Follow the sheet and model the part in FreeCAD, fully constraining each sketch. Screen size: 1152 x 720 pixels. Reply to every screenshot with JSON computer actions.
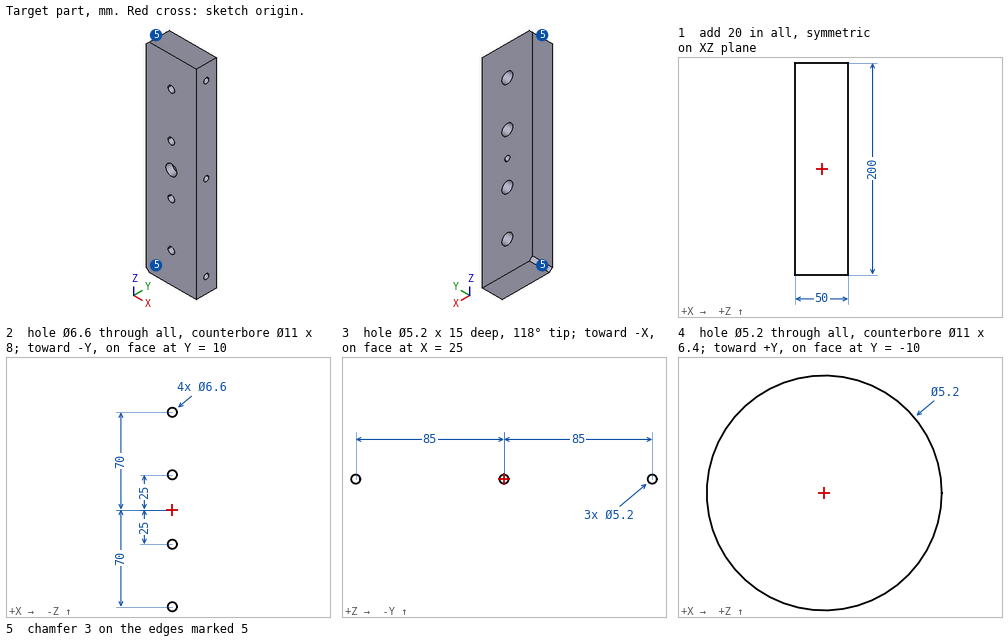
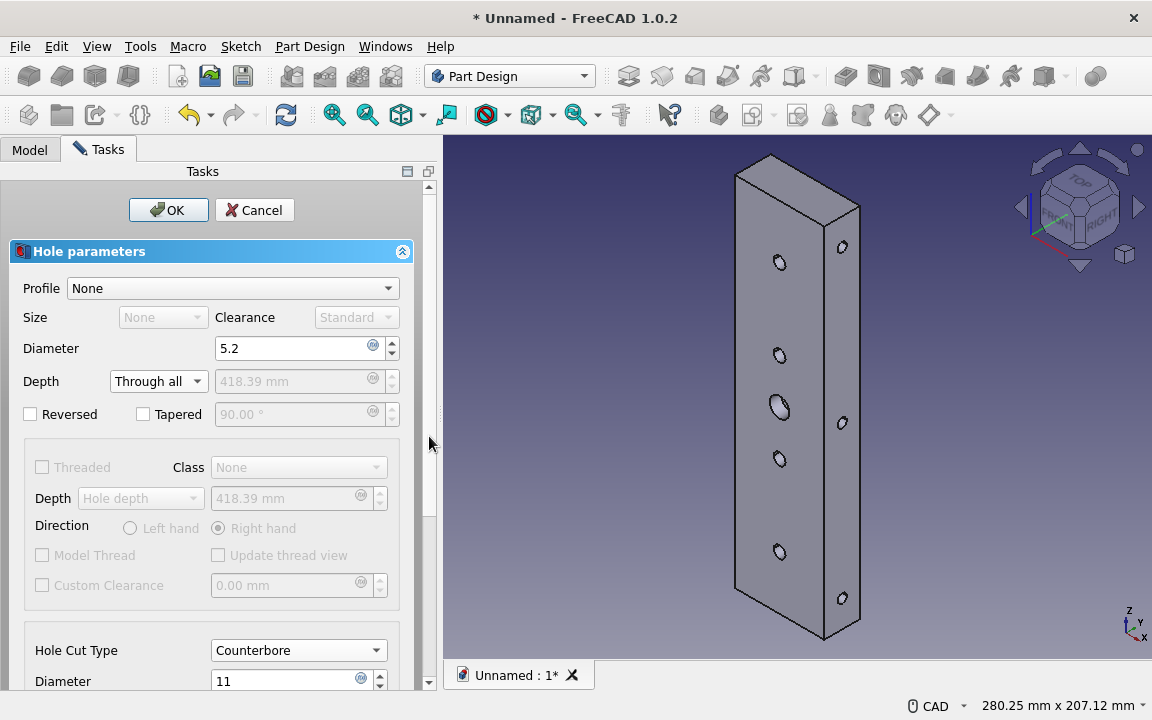
{"action": "left_click", "coordinate": [169, 210]}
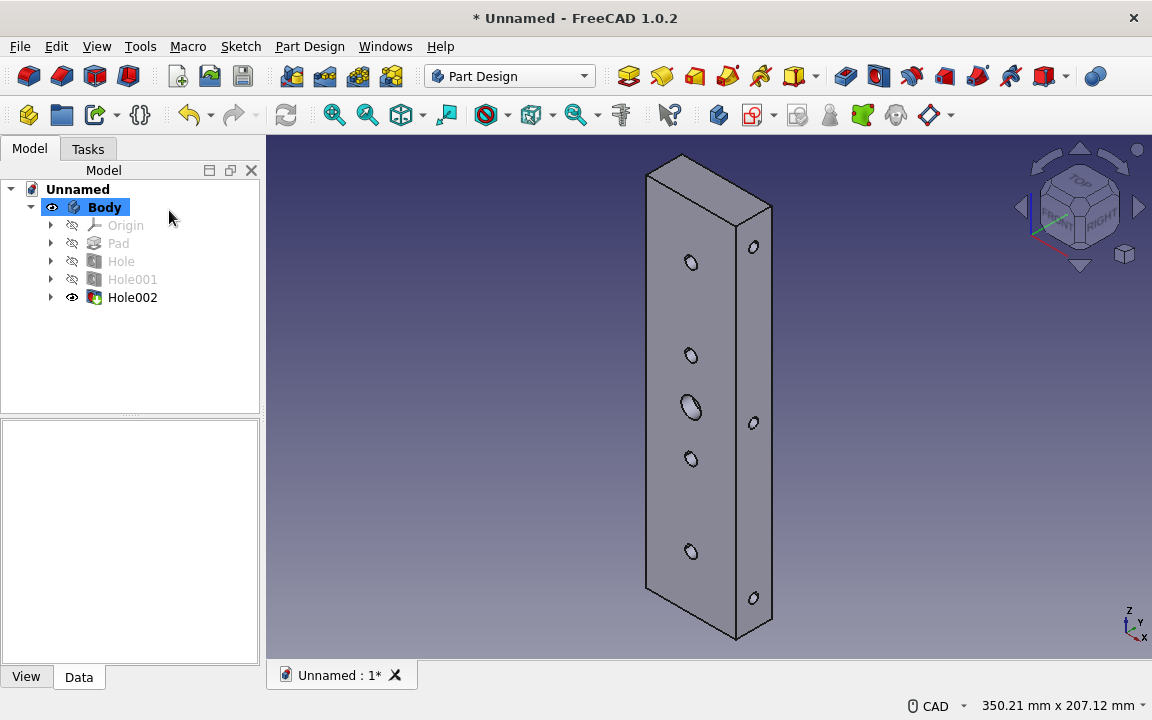
{"action": "key", "text": "2"}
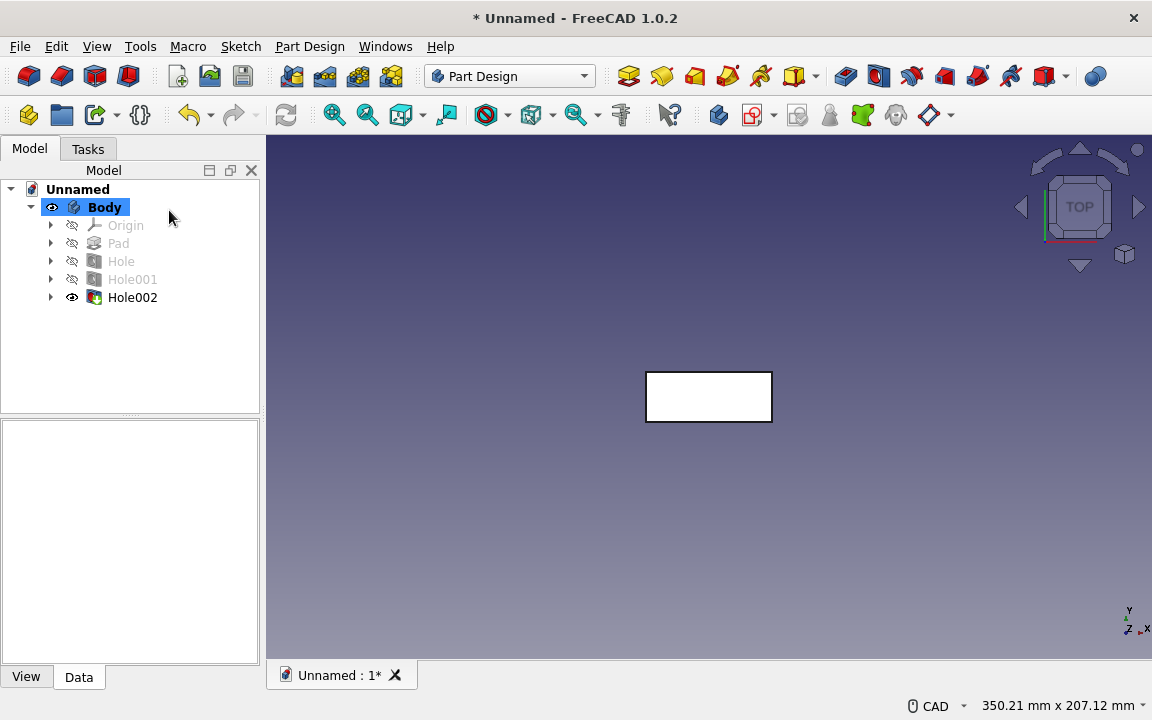
{"action": "left_click", "coordinate": [335, 116]}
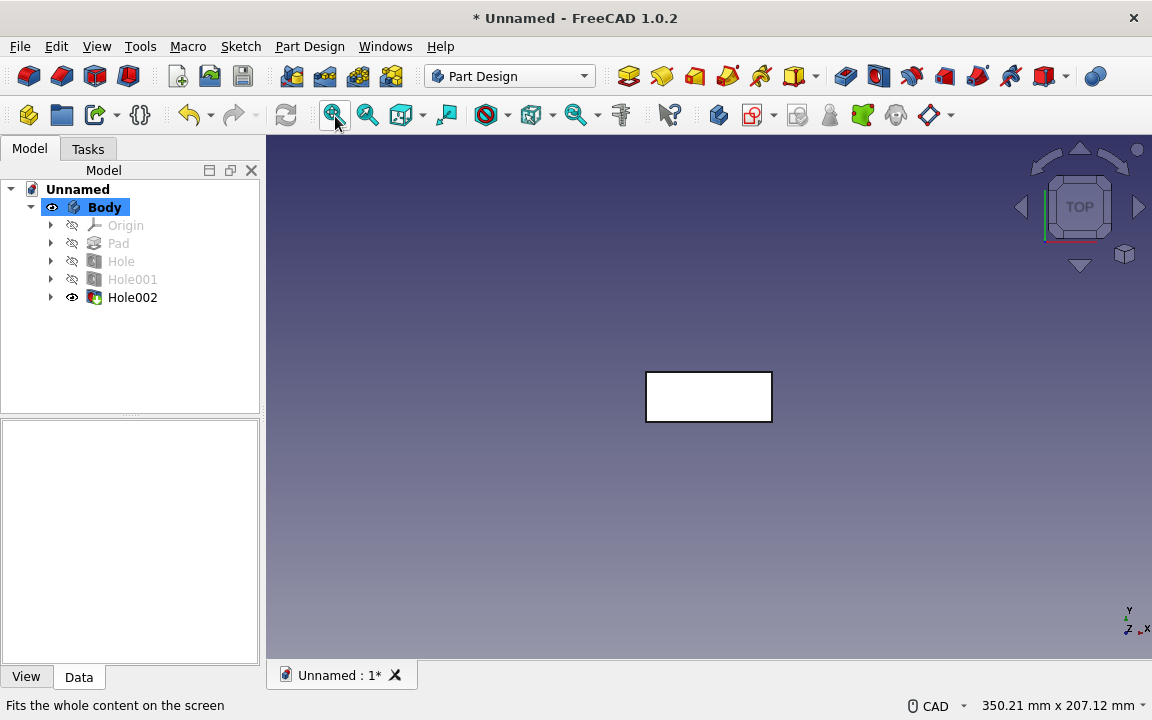
{"action": "left_click", "coordinate": [646, 396]}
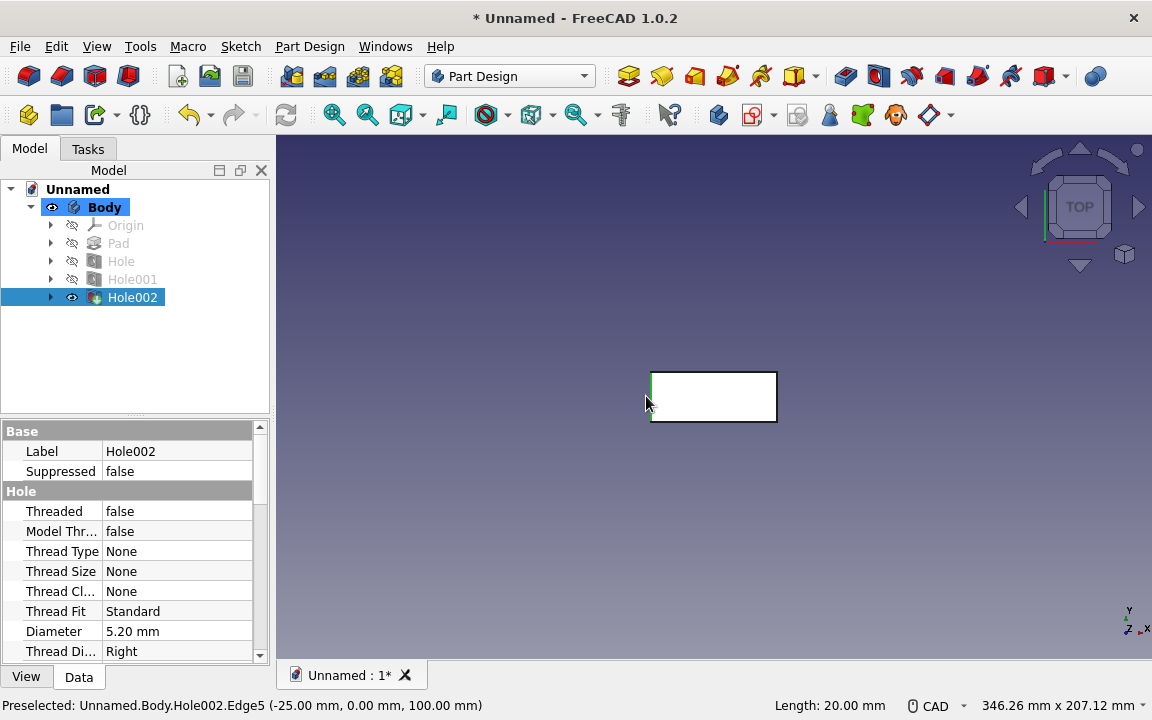
{"action": "key", "text": "0"}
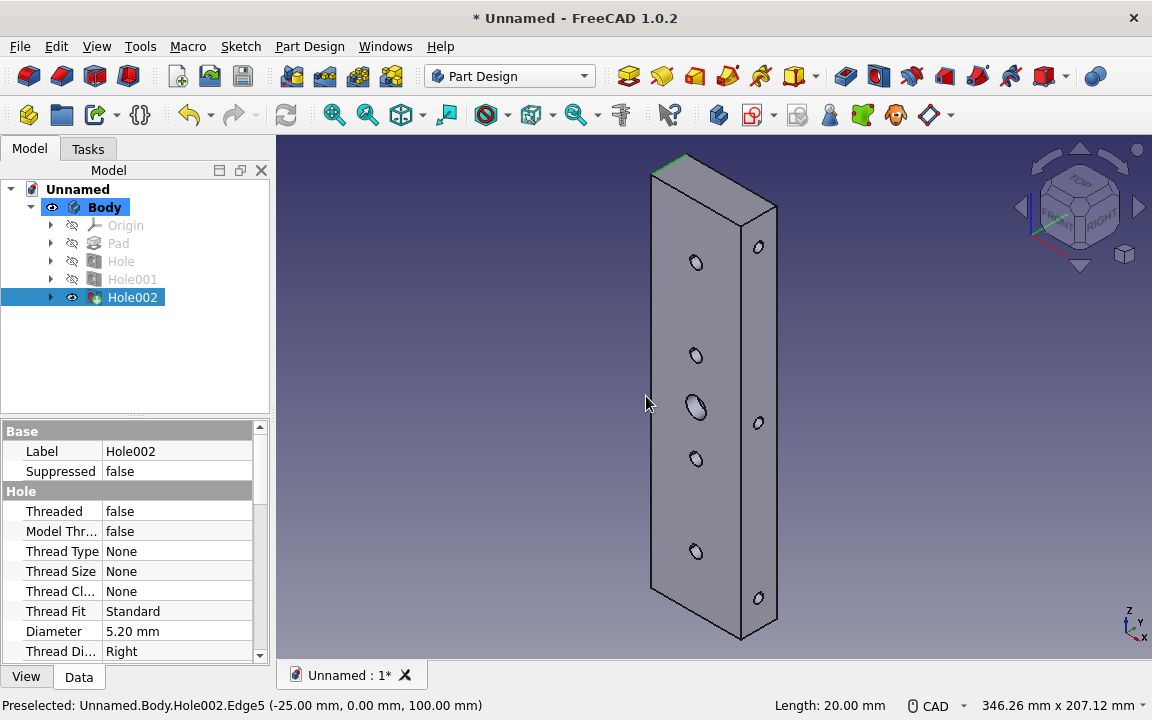
{"action": "key", "text": "1"}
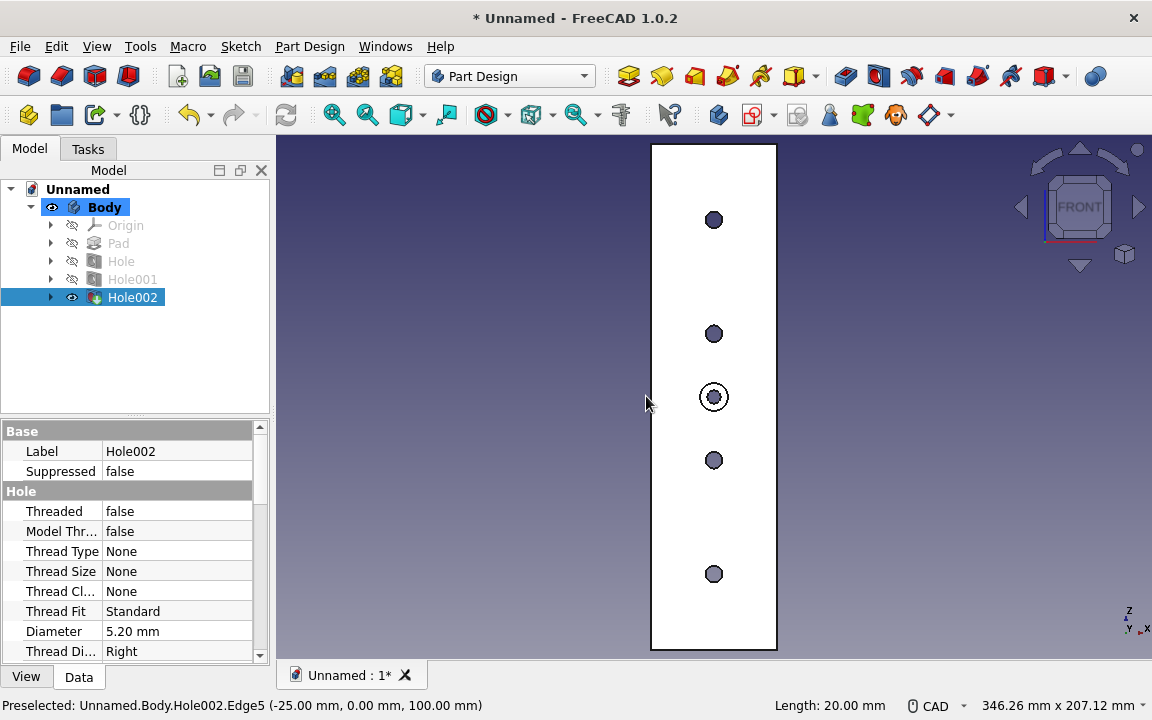
{"action": "key", "text": "3"}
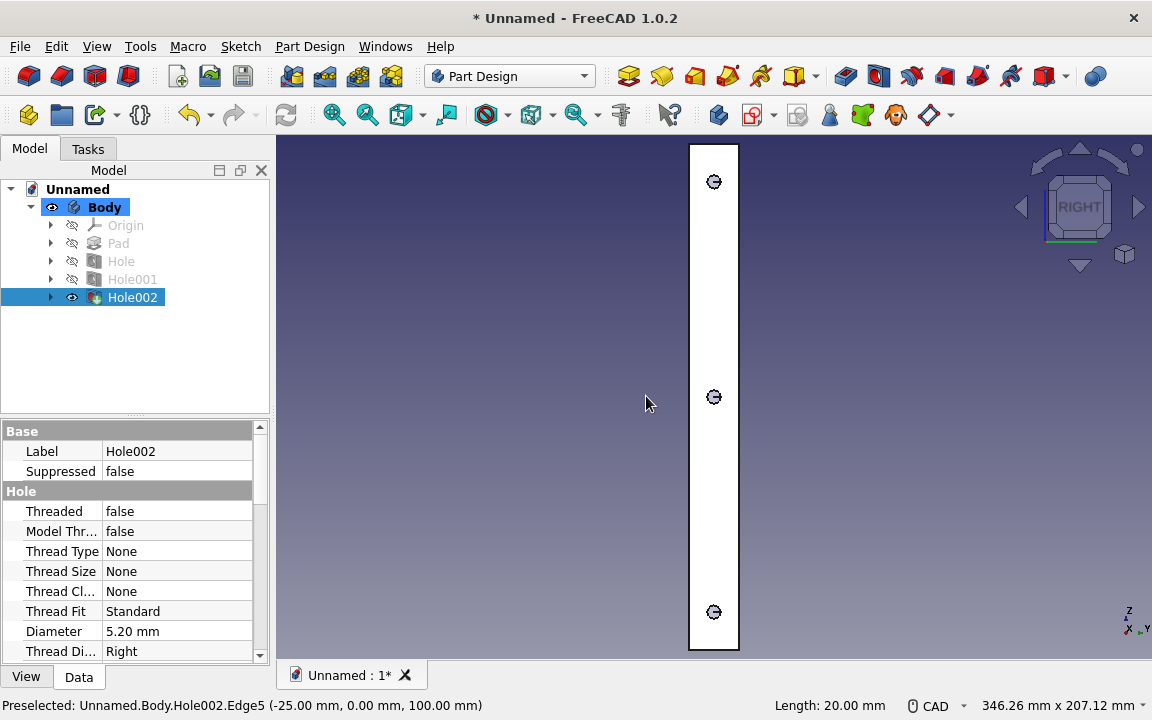
{"action": "key", "text": "5"}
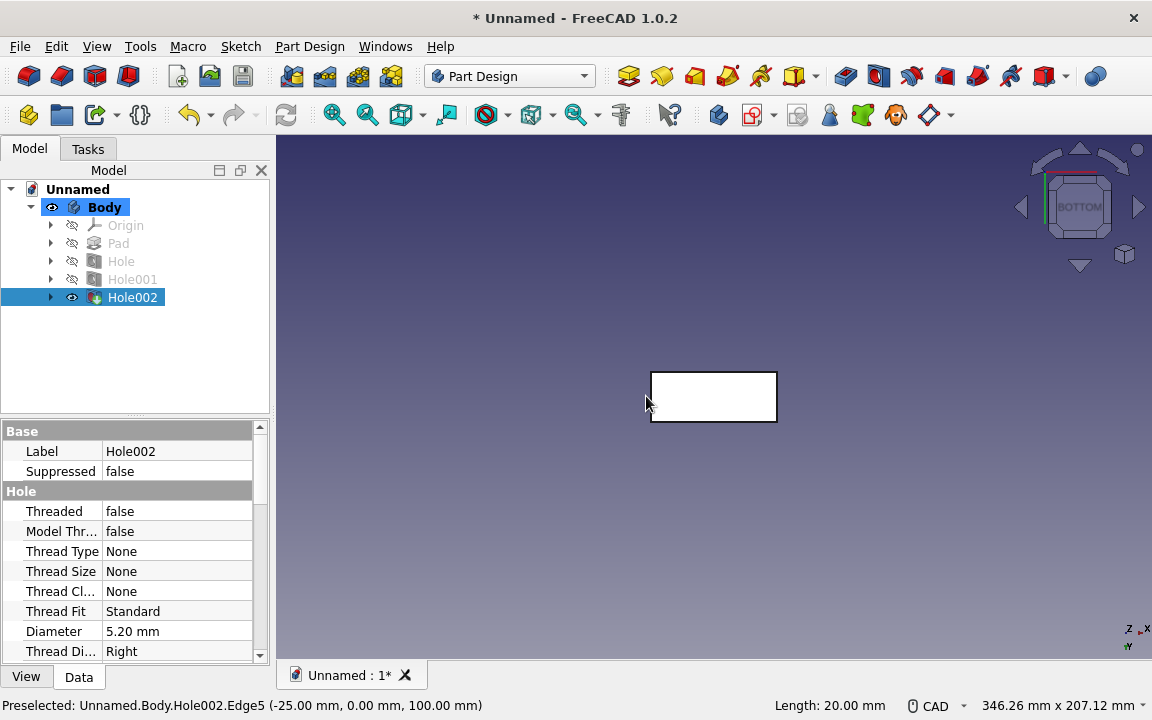
{"action": "left_click", "coordinate": [335, 116]}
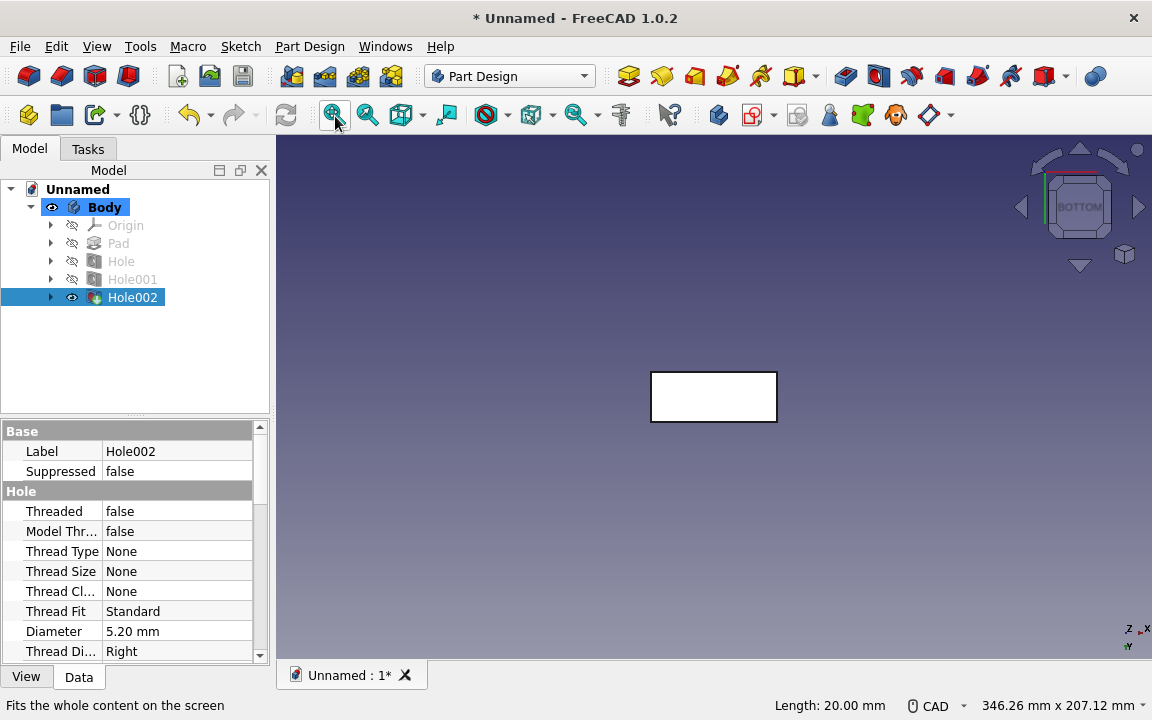
{"action": "left_click", "coordinate": [651, 396], "text": "ctrl"}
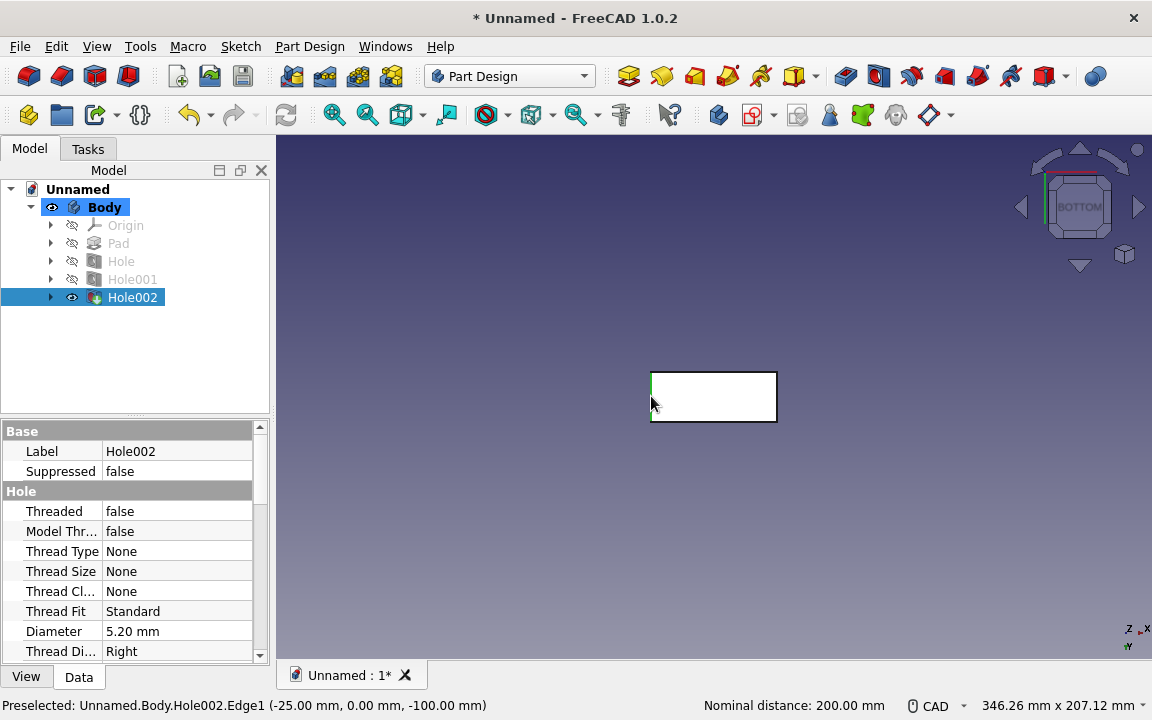
{"action": "left_click", "coordinate": [62, 76]}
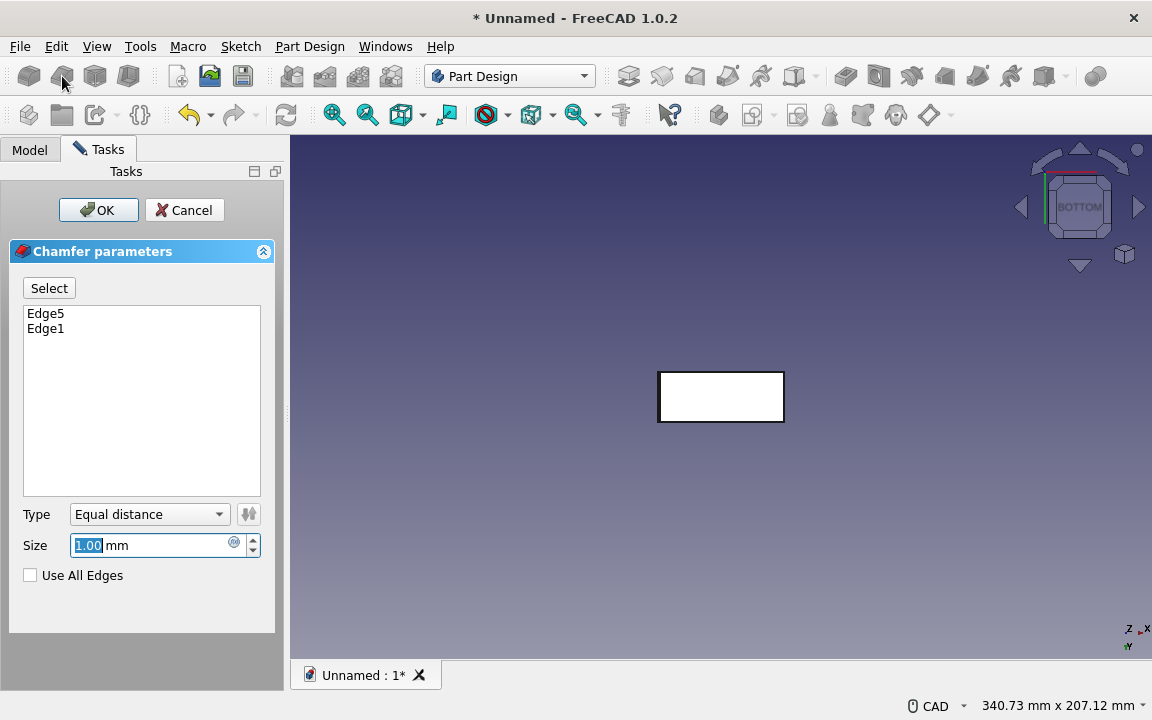
{"action": "type", "text": "3"}
{"action": "key", "text": "Tab"}